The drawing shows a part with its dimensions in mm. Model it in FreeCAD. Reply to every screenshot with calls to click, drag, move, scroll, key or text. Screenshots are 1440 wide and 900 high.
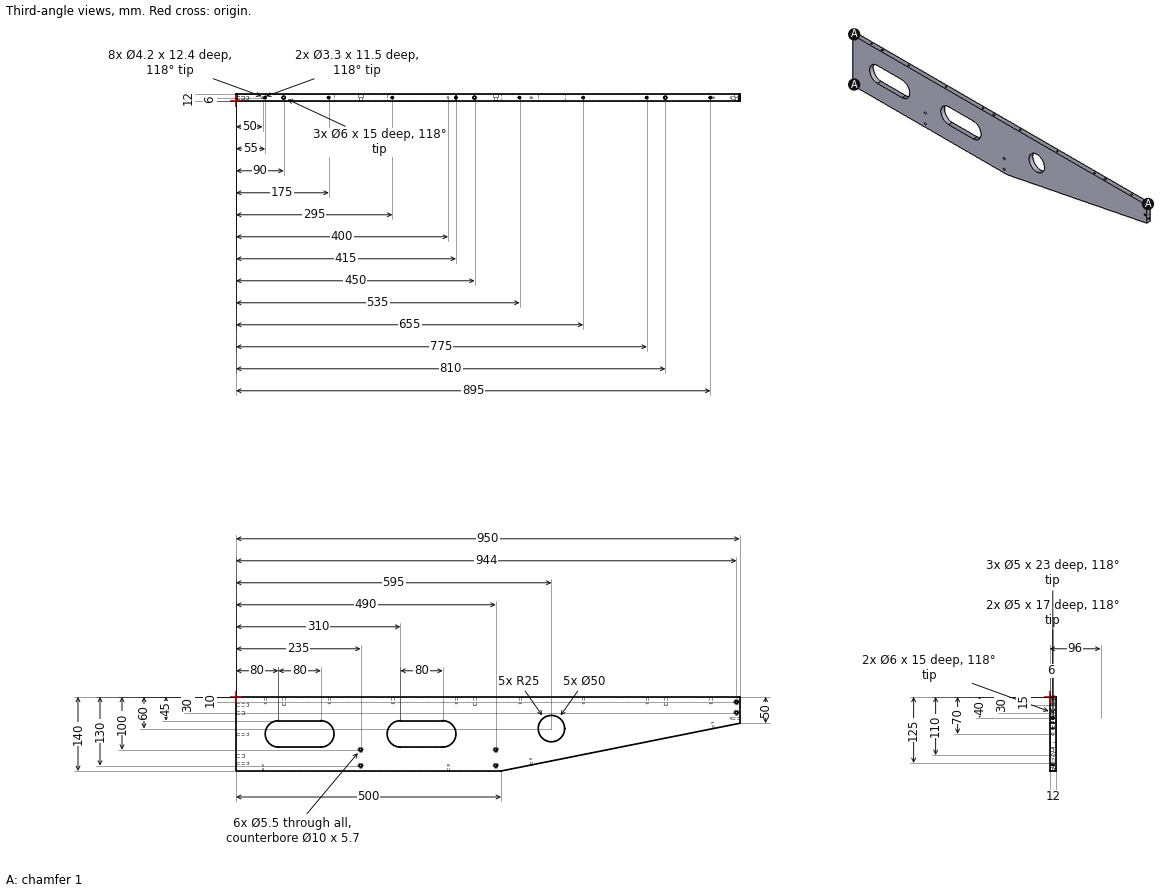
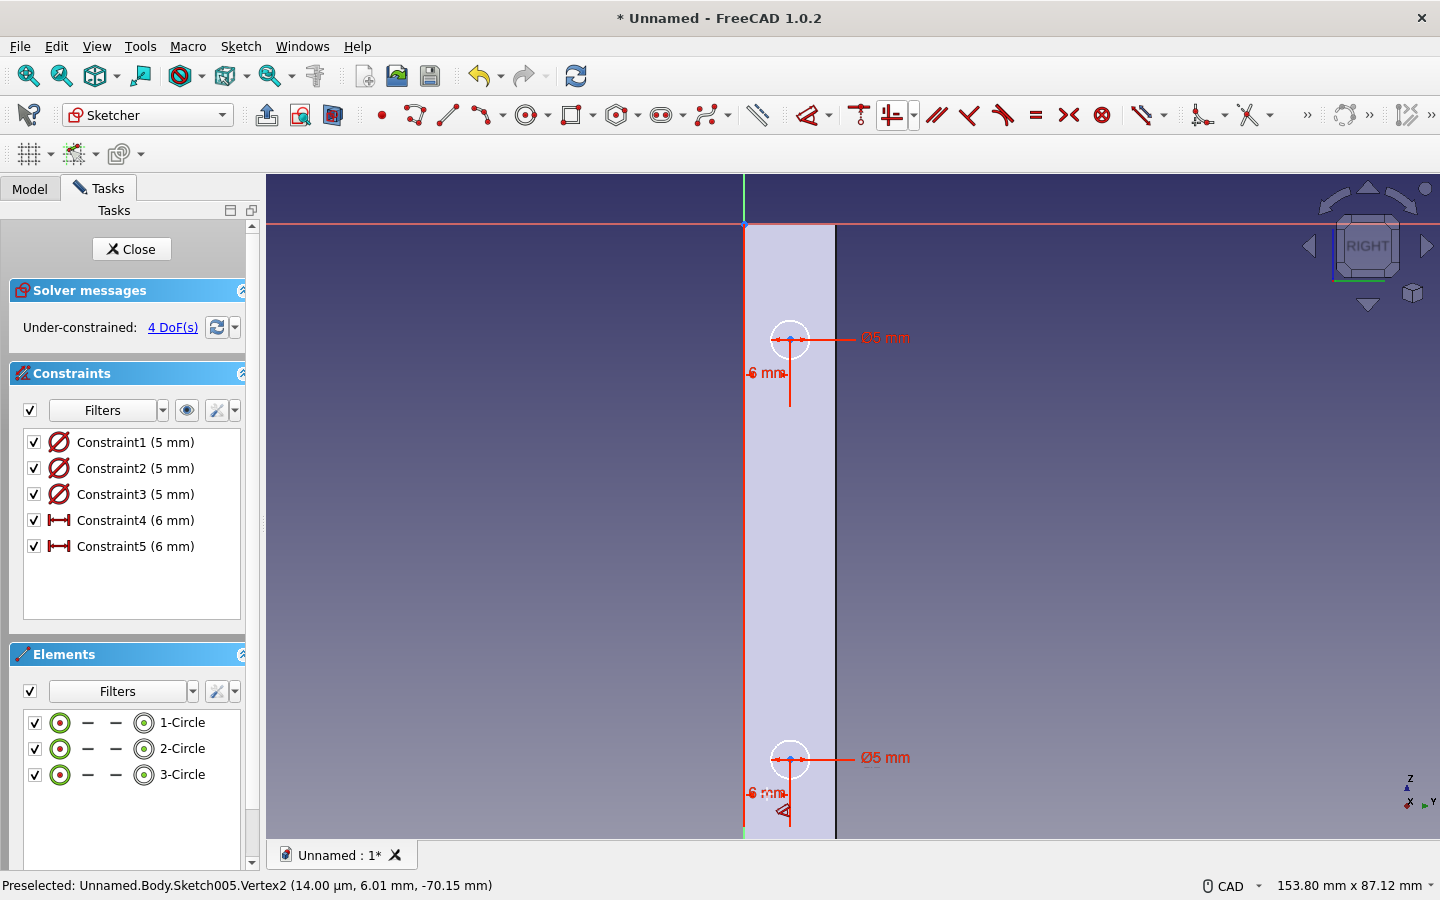
scroll(791, 340, down, 4)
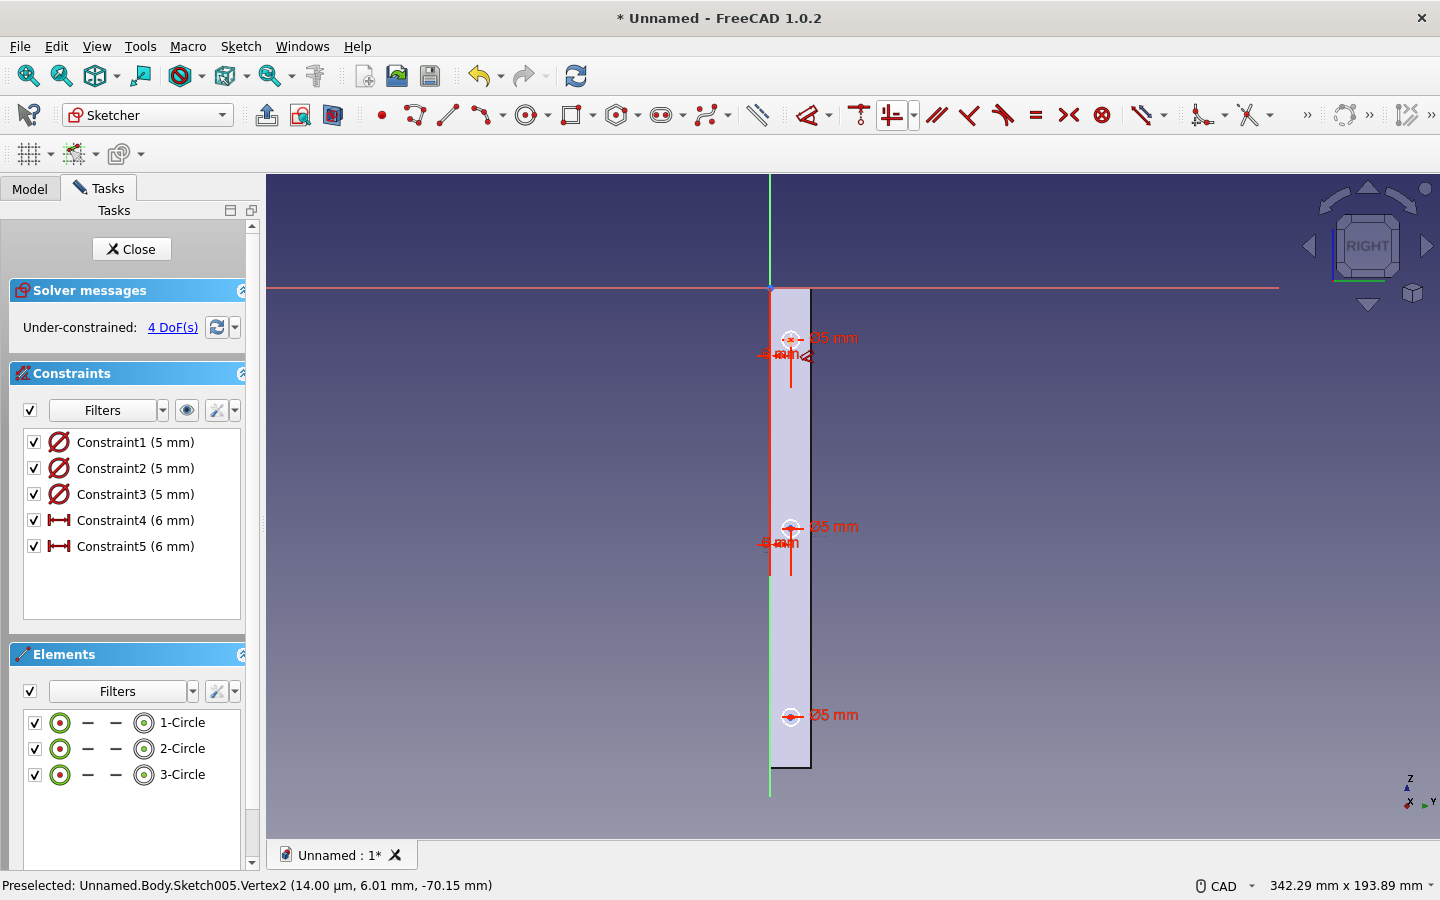
scroll(791, 717, up, 4)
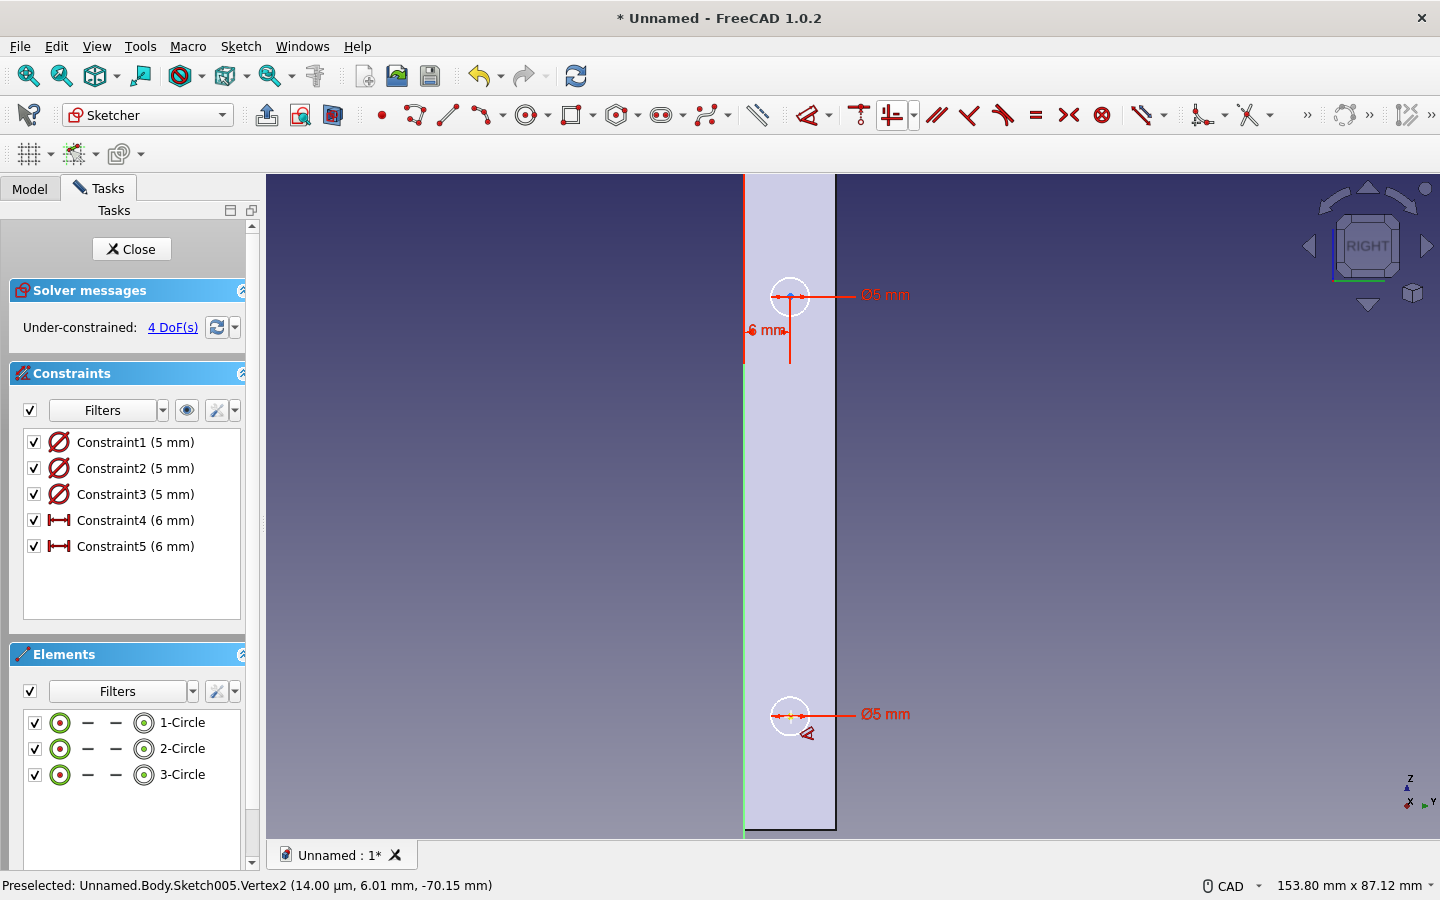
click(790, 716)
click(767, 750)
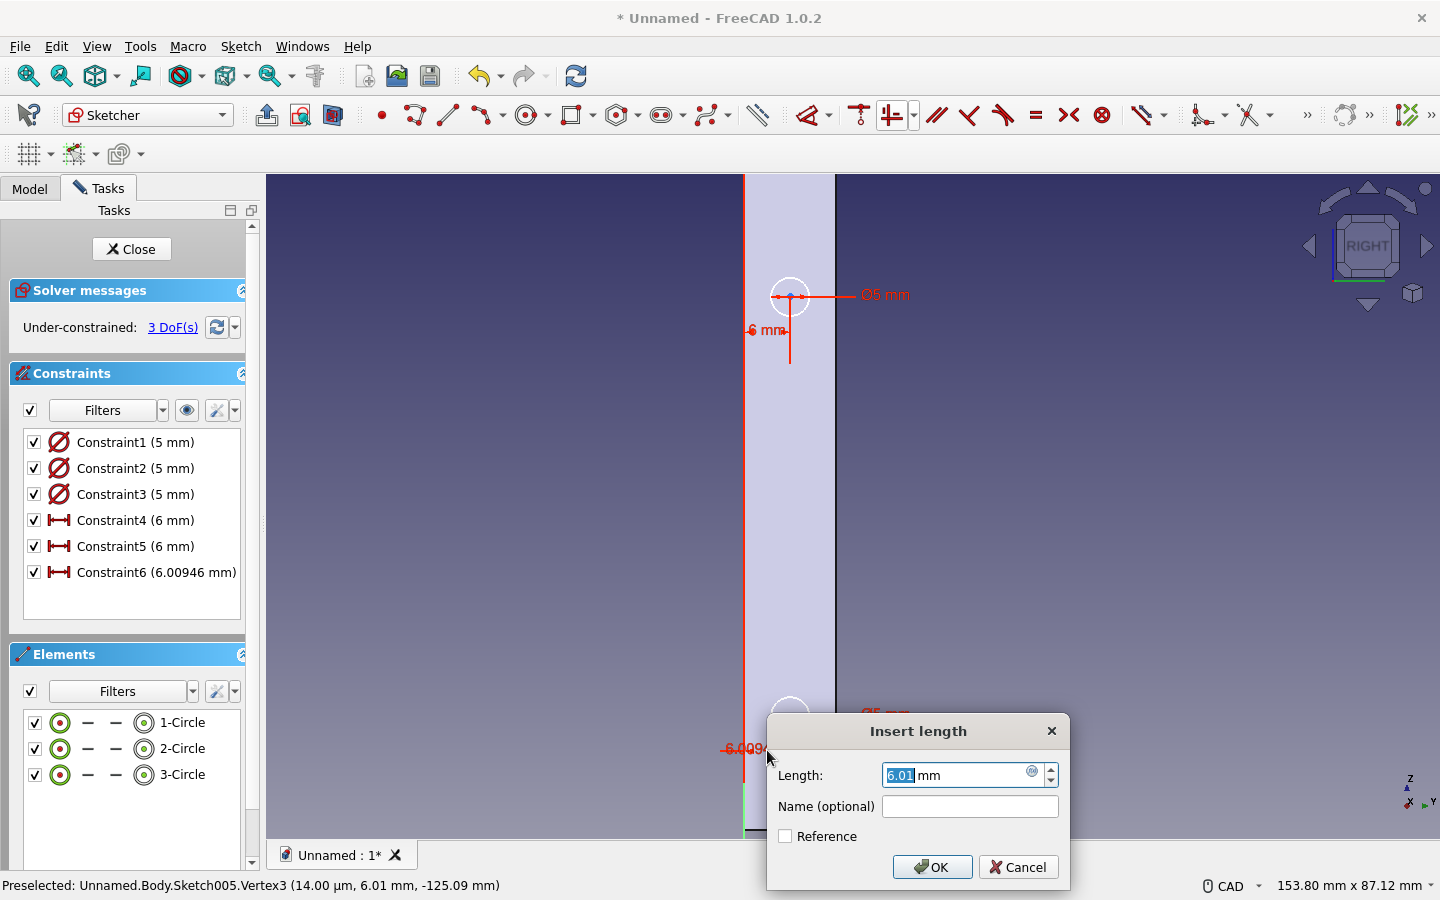
text(6)
key(Return)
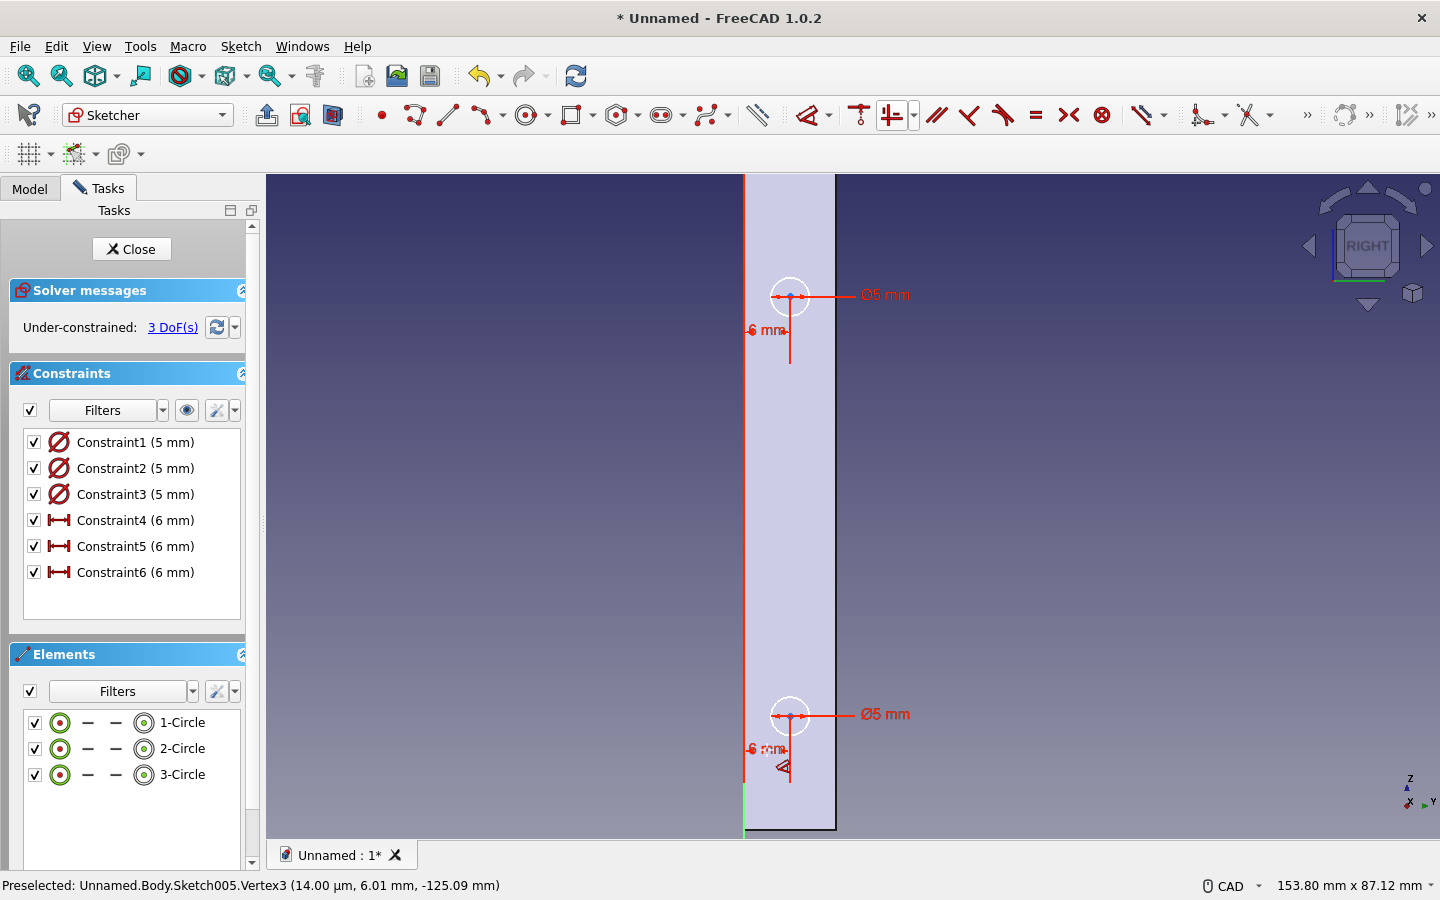
scroll(791, 717, down, 4)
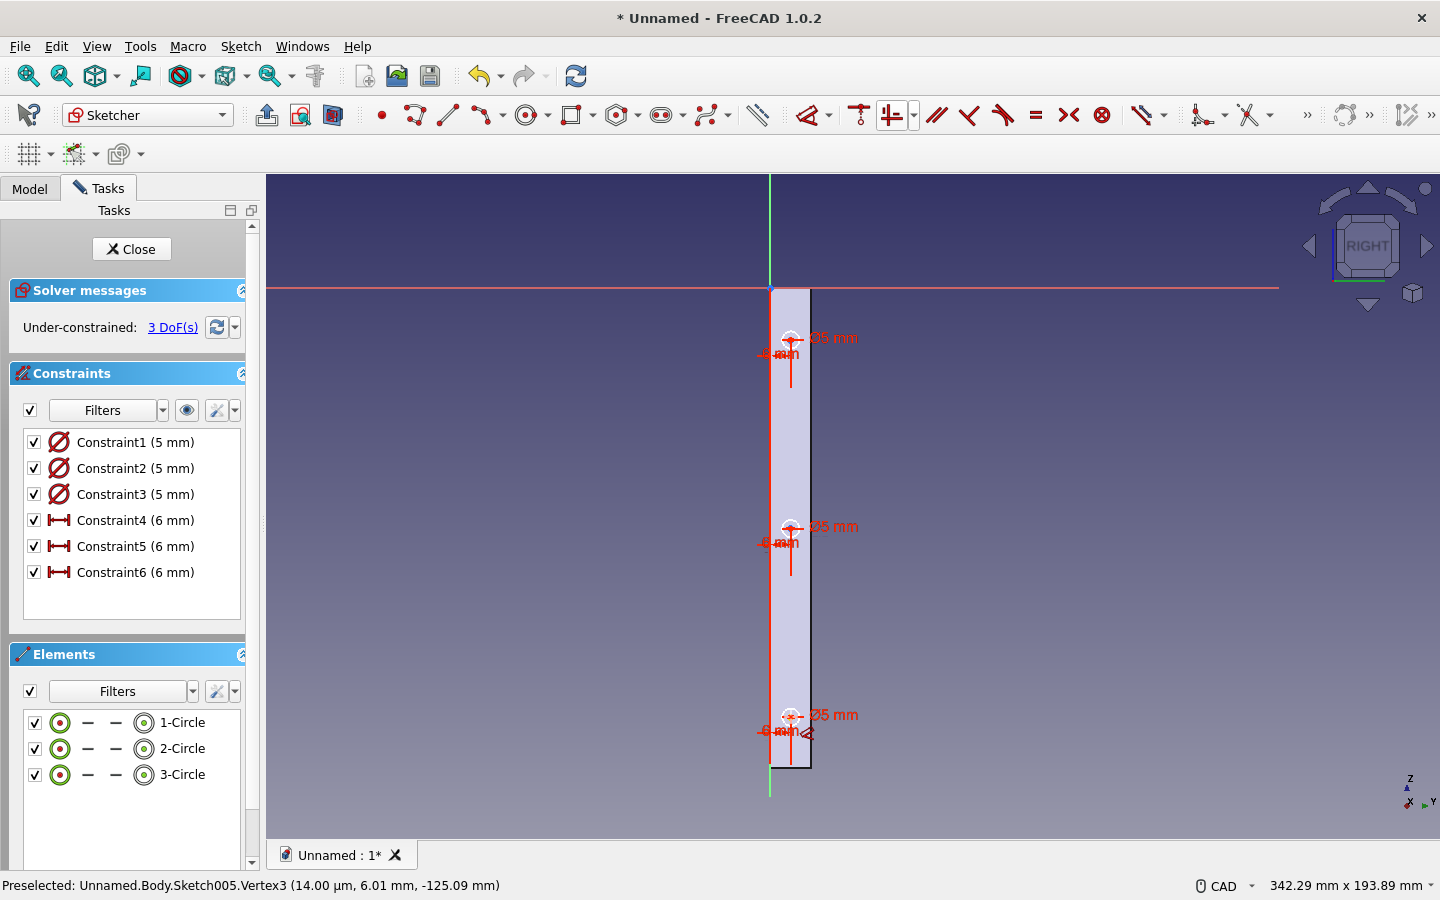
click(791, 340)
click(736, 314)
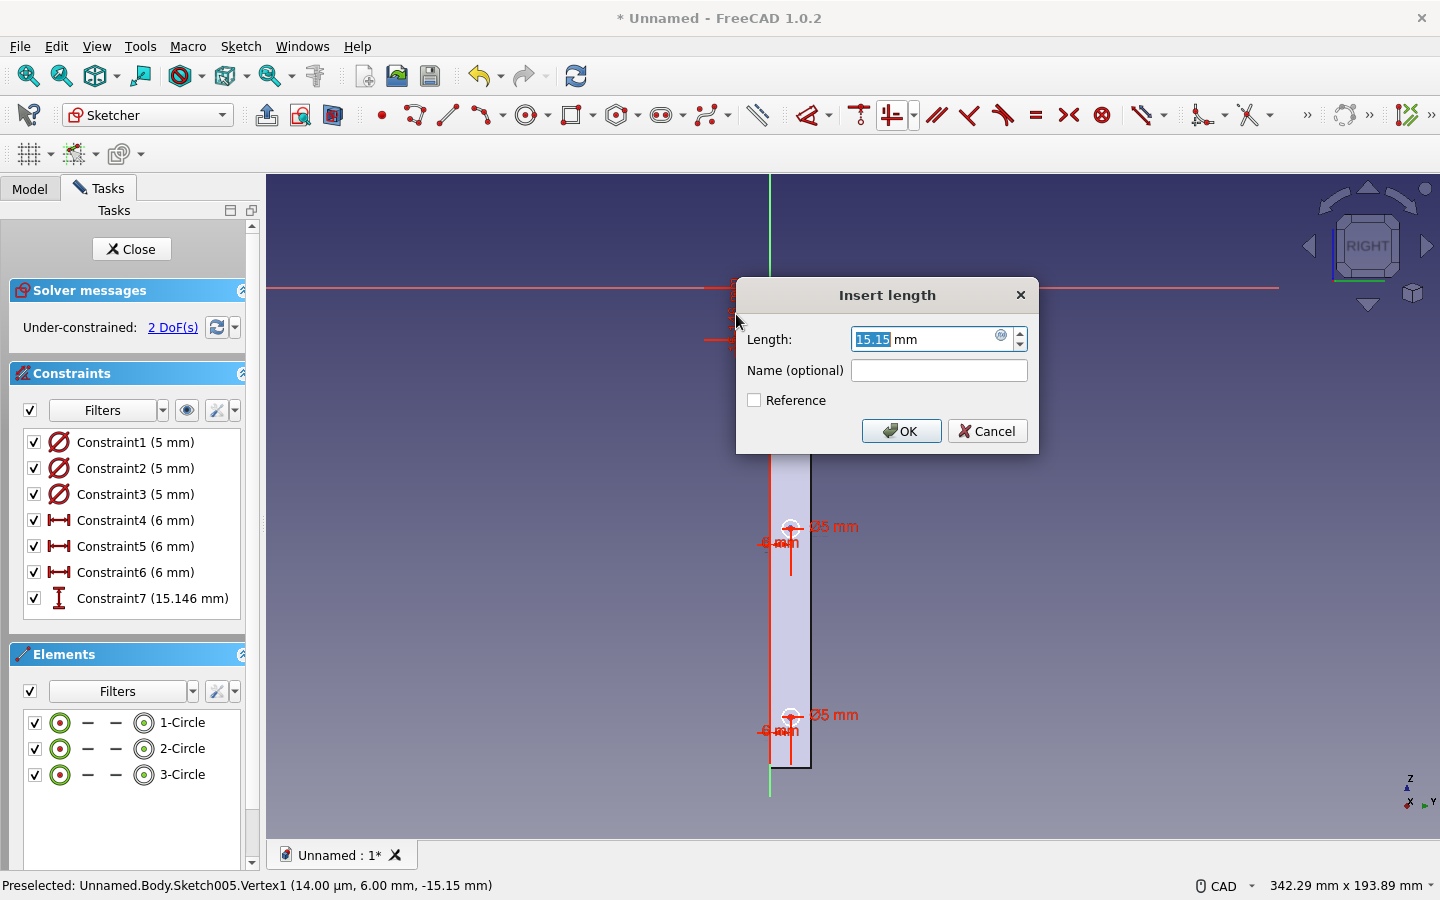
text(15)
key(Return)